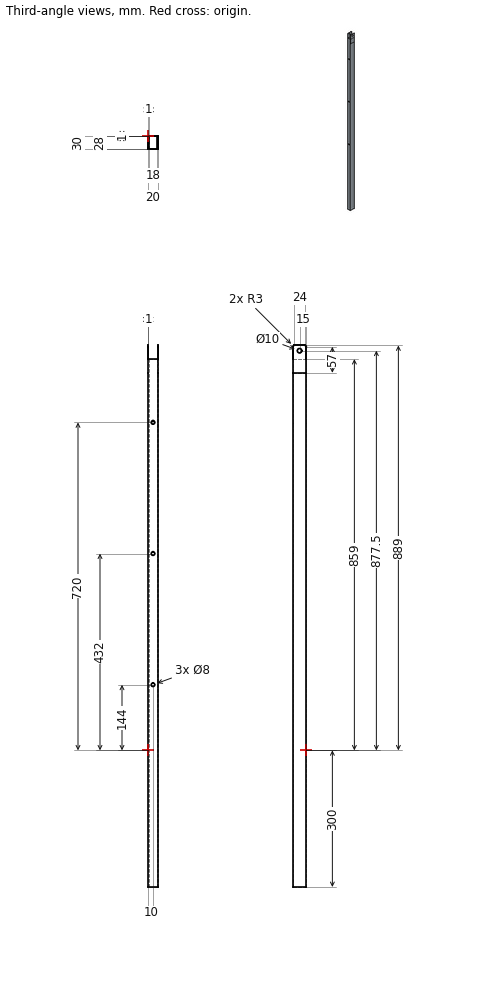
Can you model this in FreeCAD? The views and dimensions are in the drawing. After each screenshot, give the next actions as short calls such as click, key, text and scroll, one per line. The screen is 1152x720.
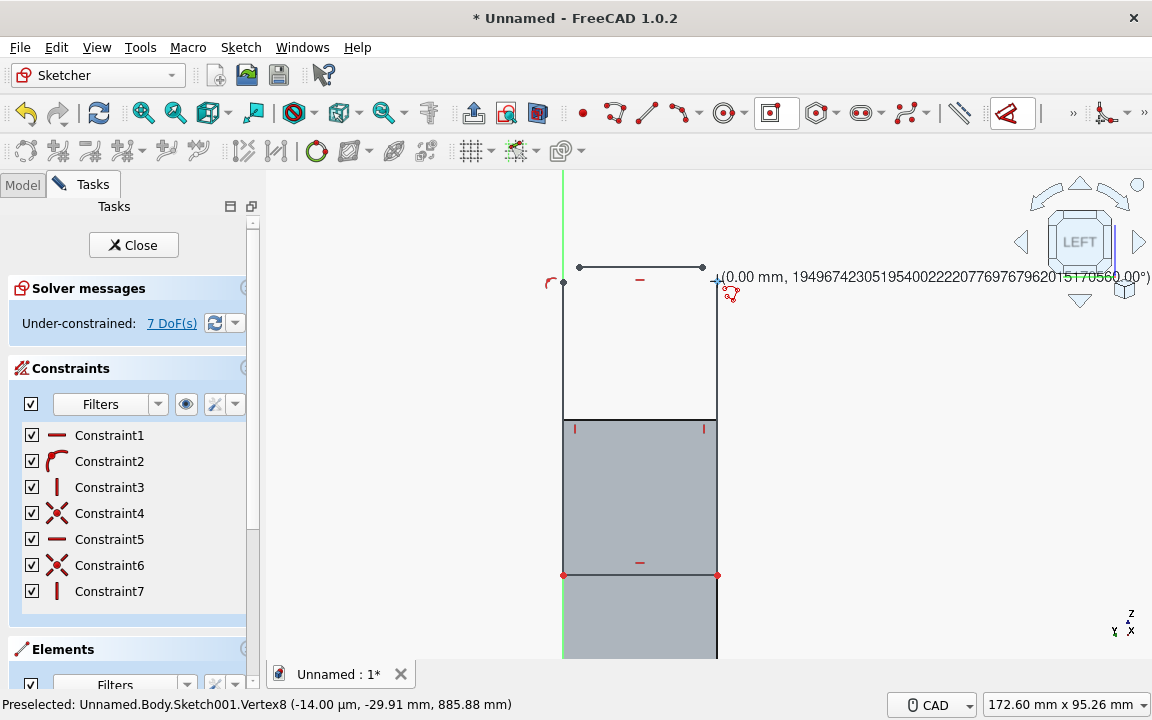
key(g)
key(3)
key(a)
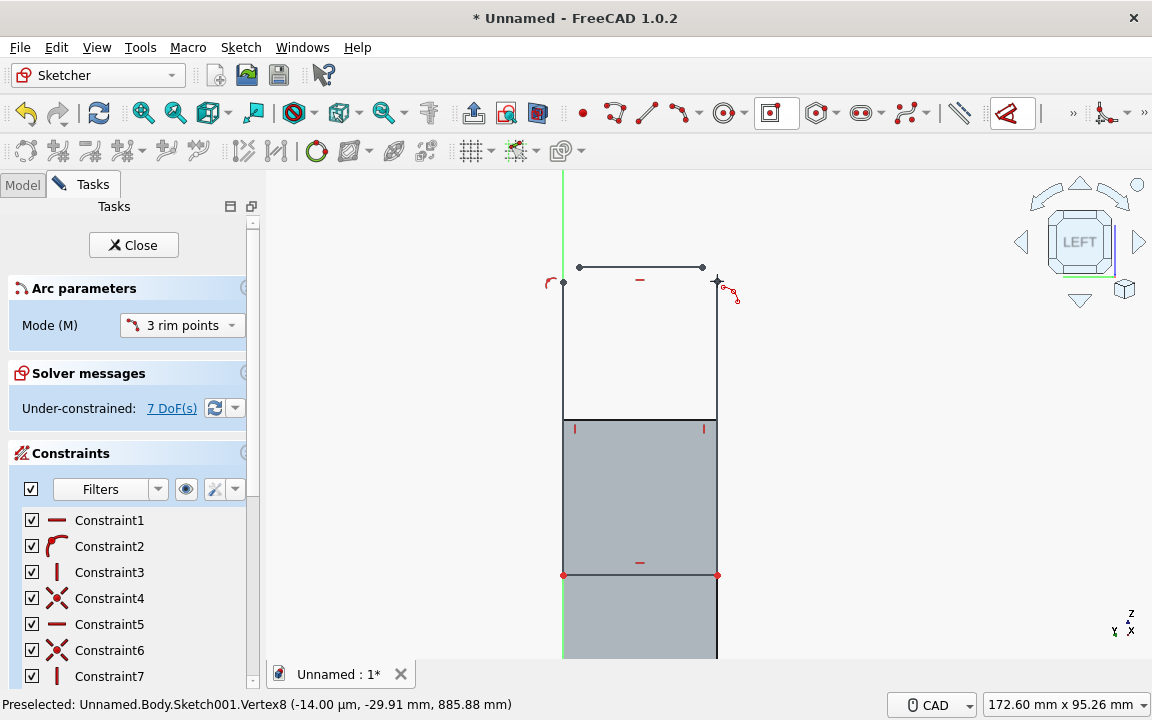
click(579, 267)
click(563, 282)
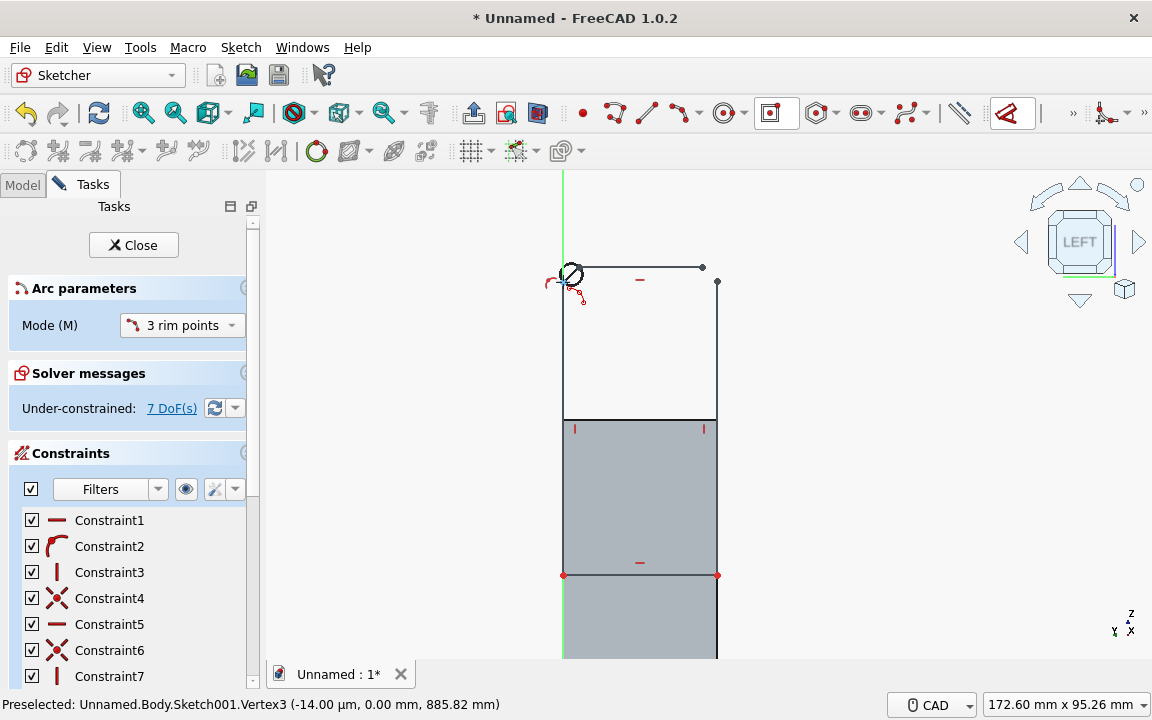
scroll(568, 271, up, 7)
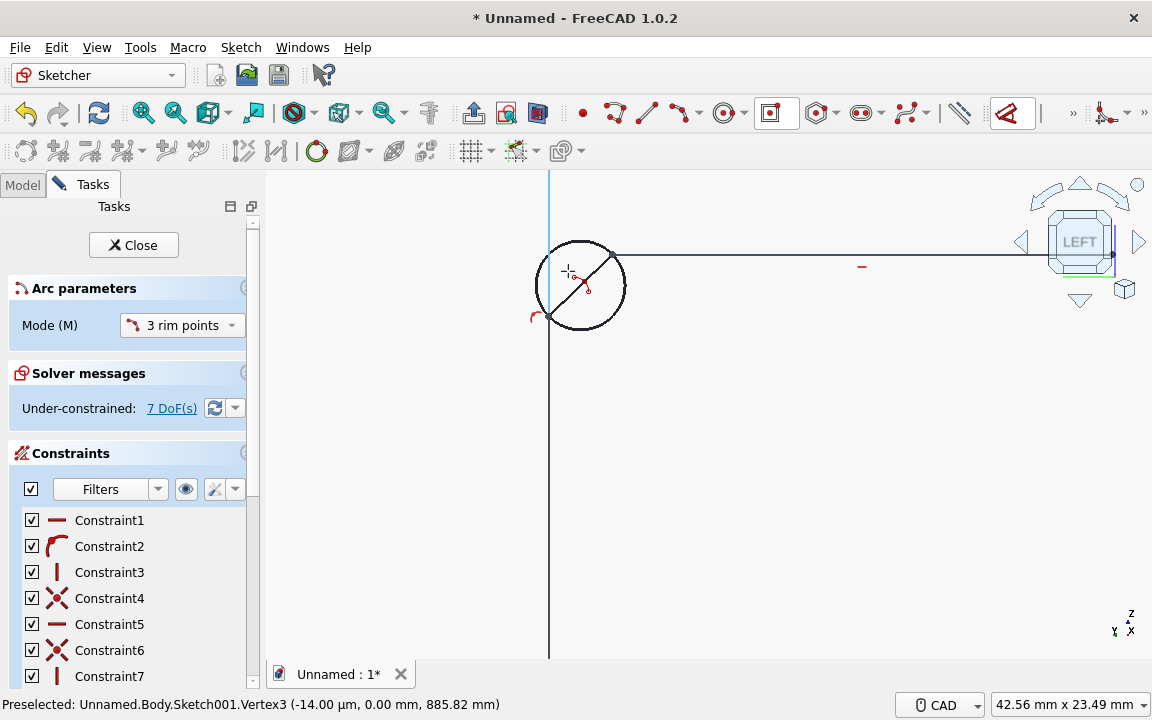
click(567, 268)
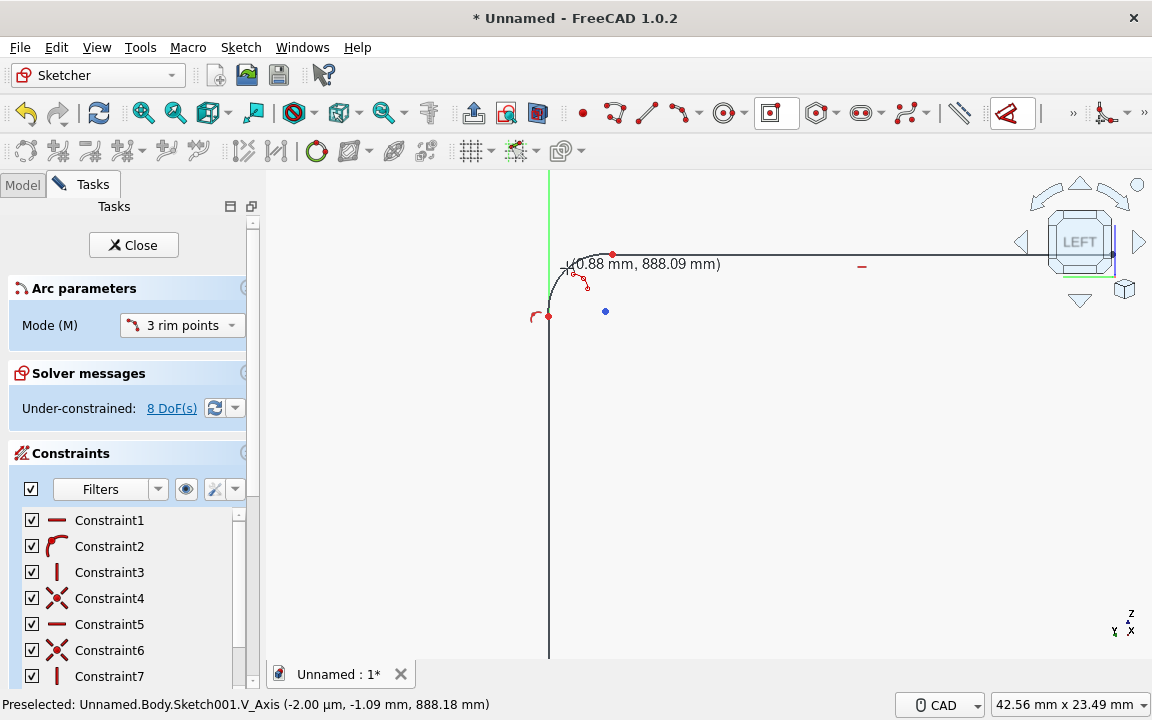
scroll(568, 264, down, 7)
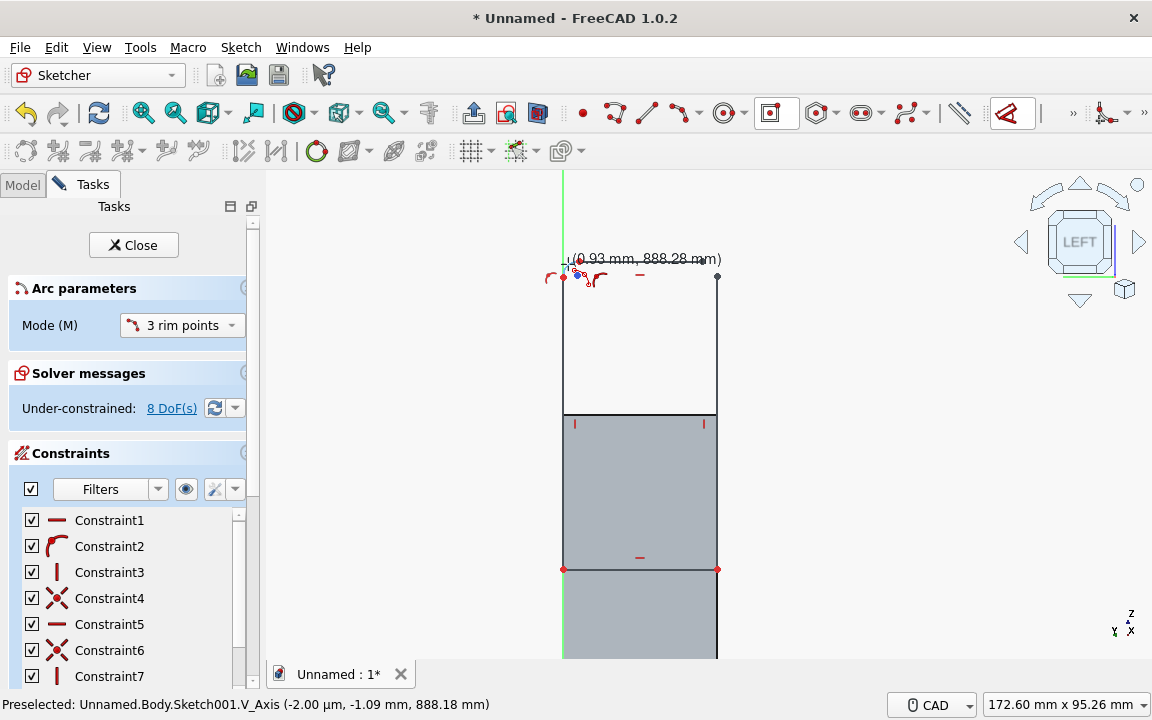
click(717, 277)
click(702, 262)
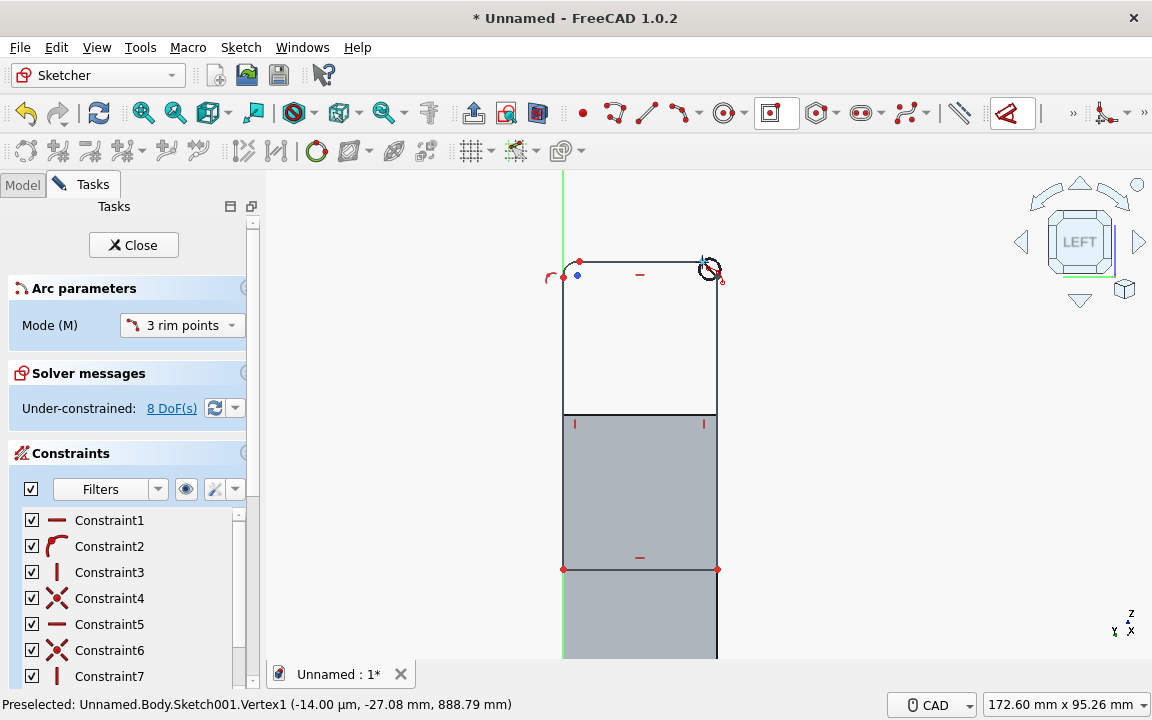
scroll(713, 265, up, 7)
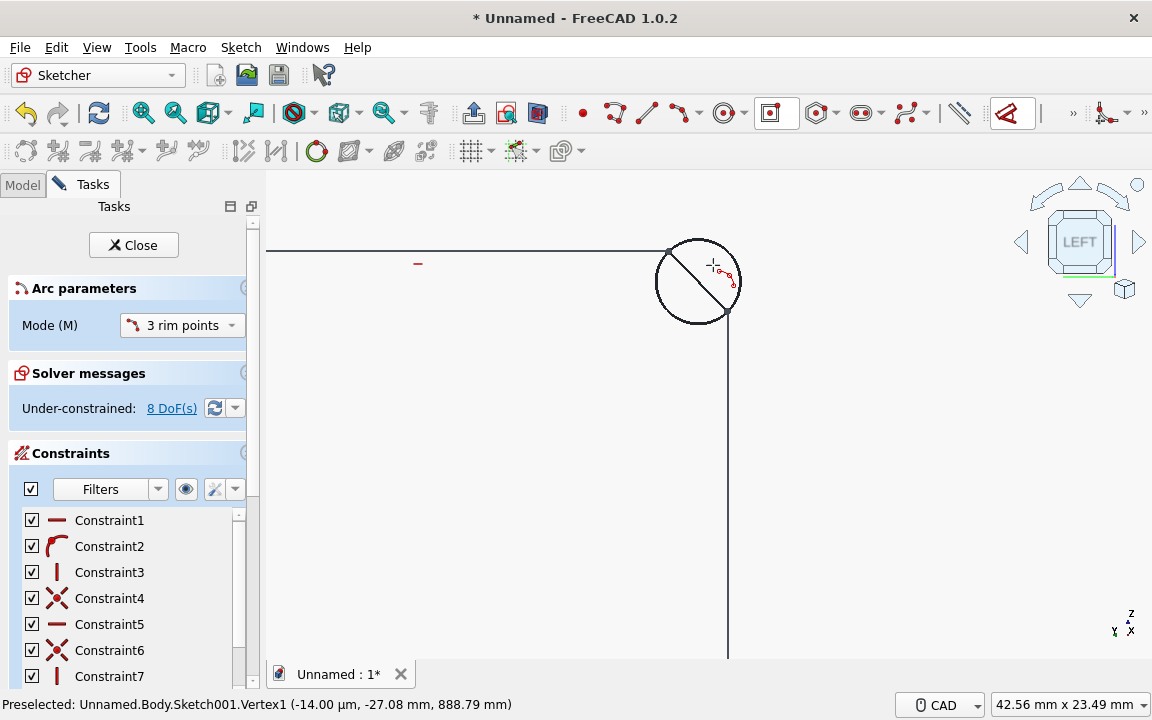
click(711, 265)
key(Escape)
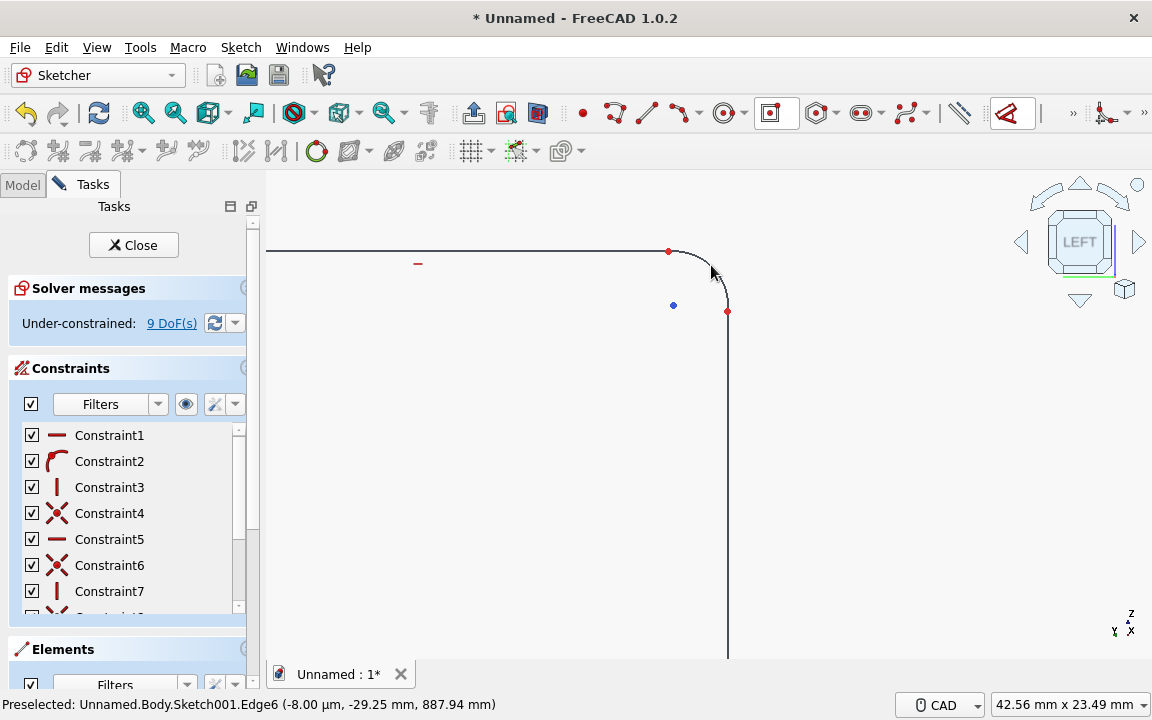
scroll(714, 265, down, 7)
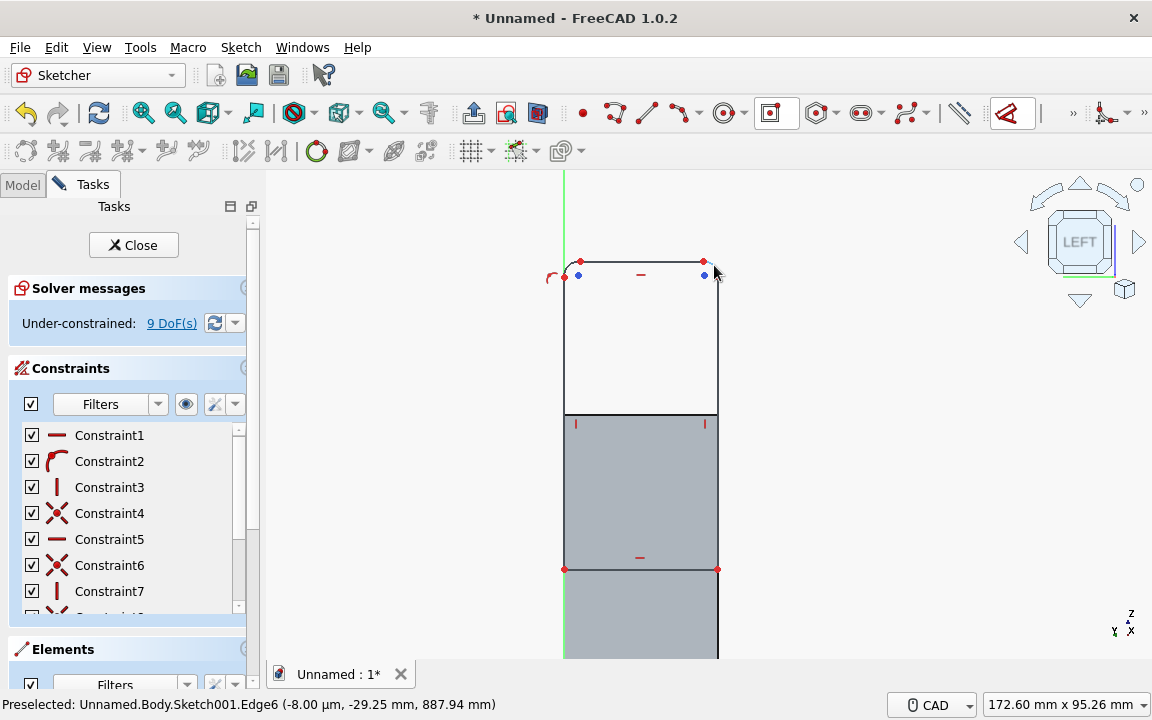
click(666, 262)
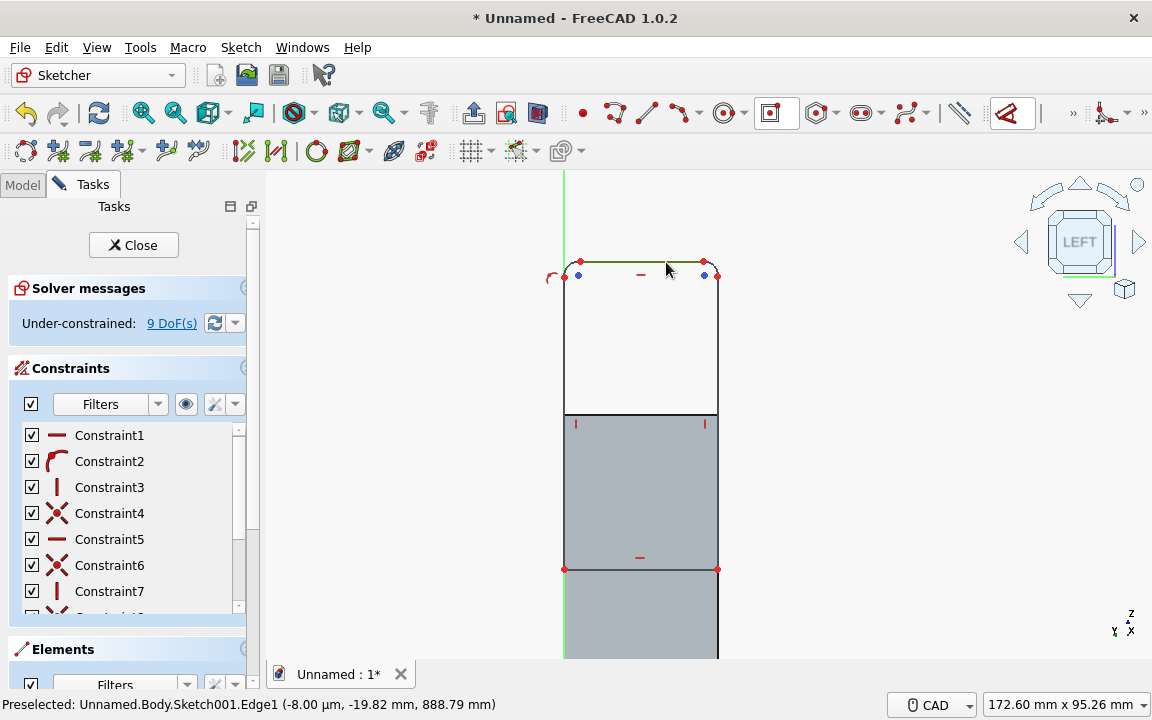
scroll(566, 270, up, 4)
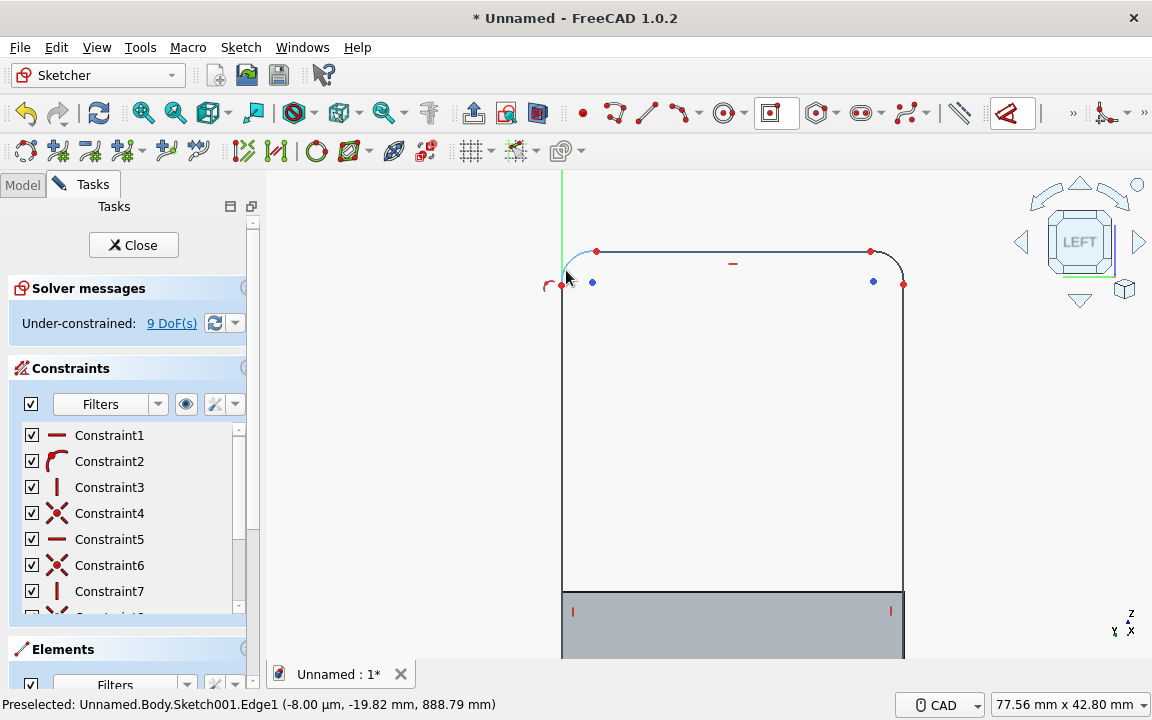
click(565, 269)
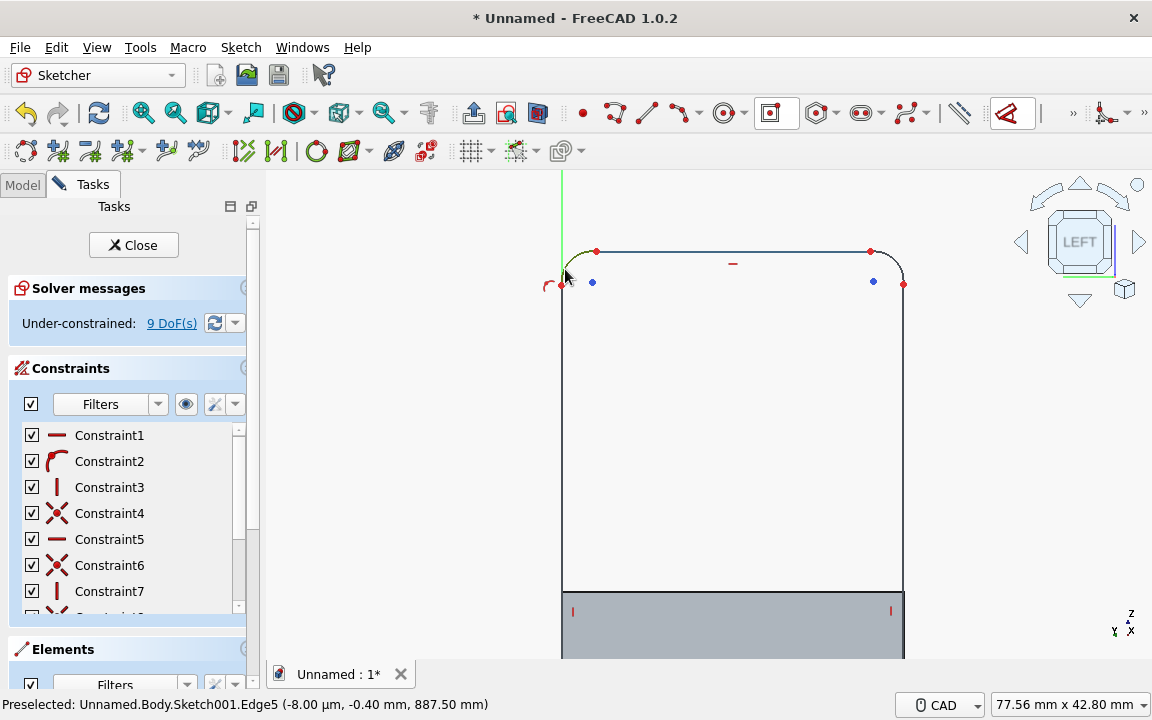
key(t)